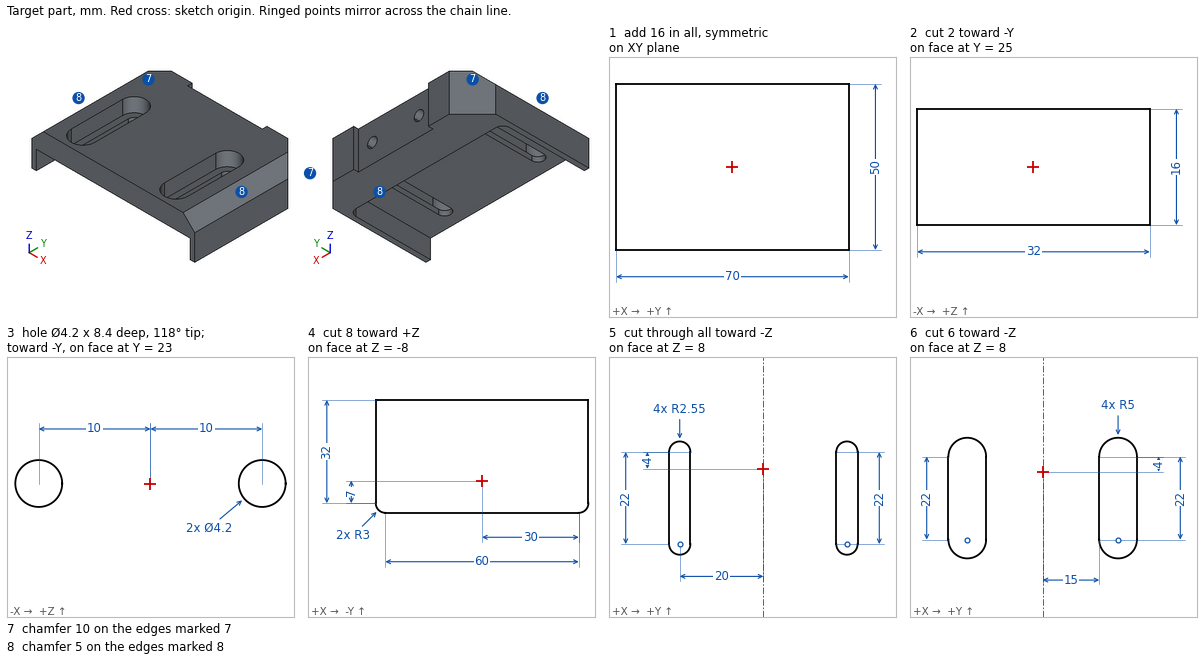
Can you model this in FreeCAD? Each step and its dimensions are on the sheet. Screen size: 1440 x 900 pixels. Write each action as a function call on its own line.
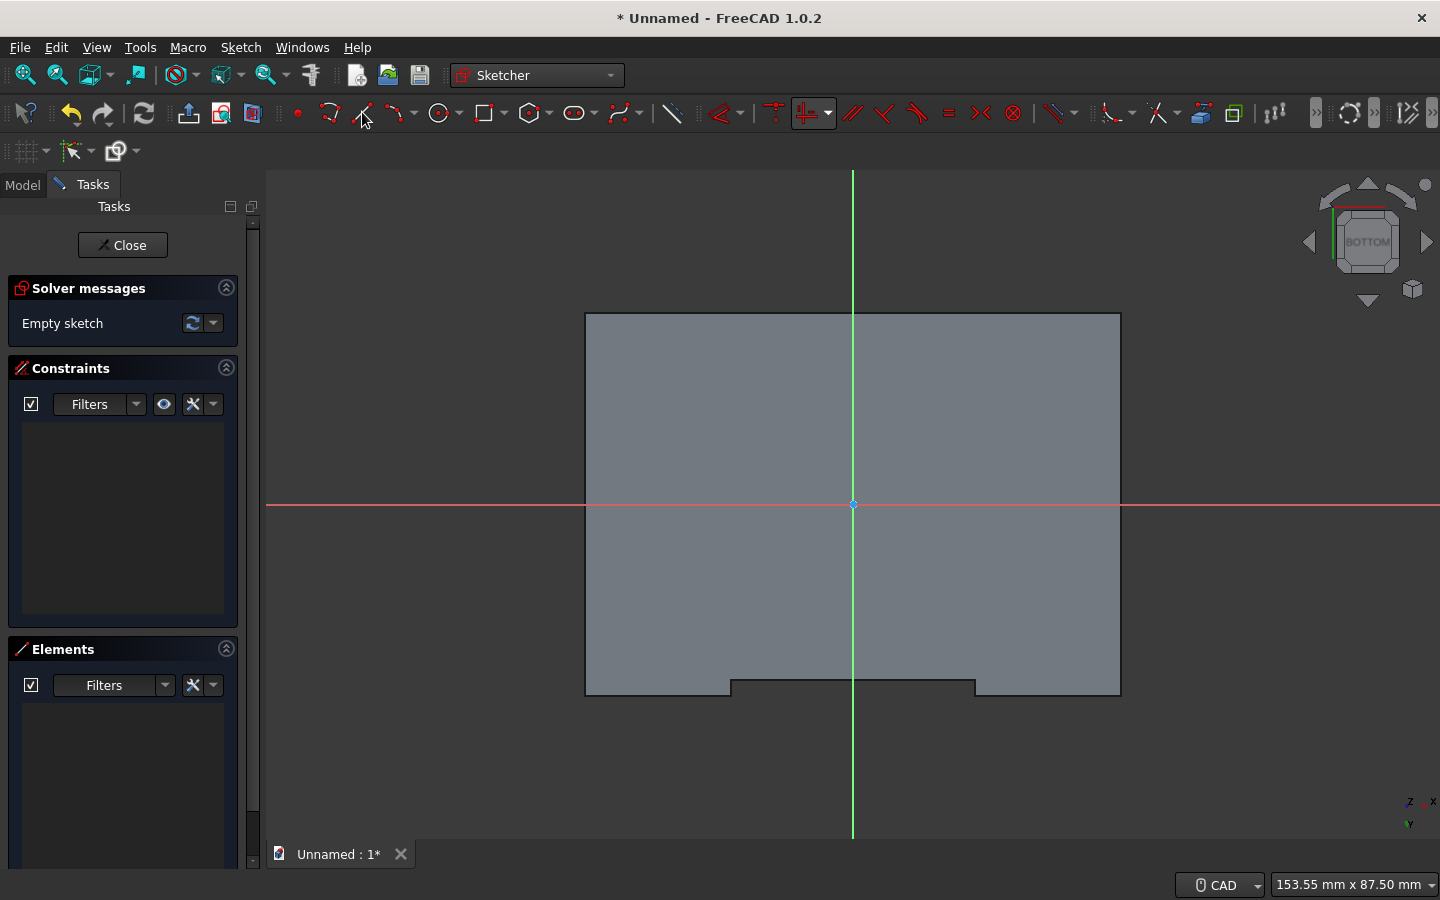
scroll(992, 331, up, 2)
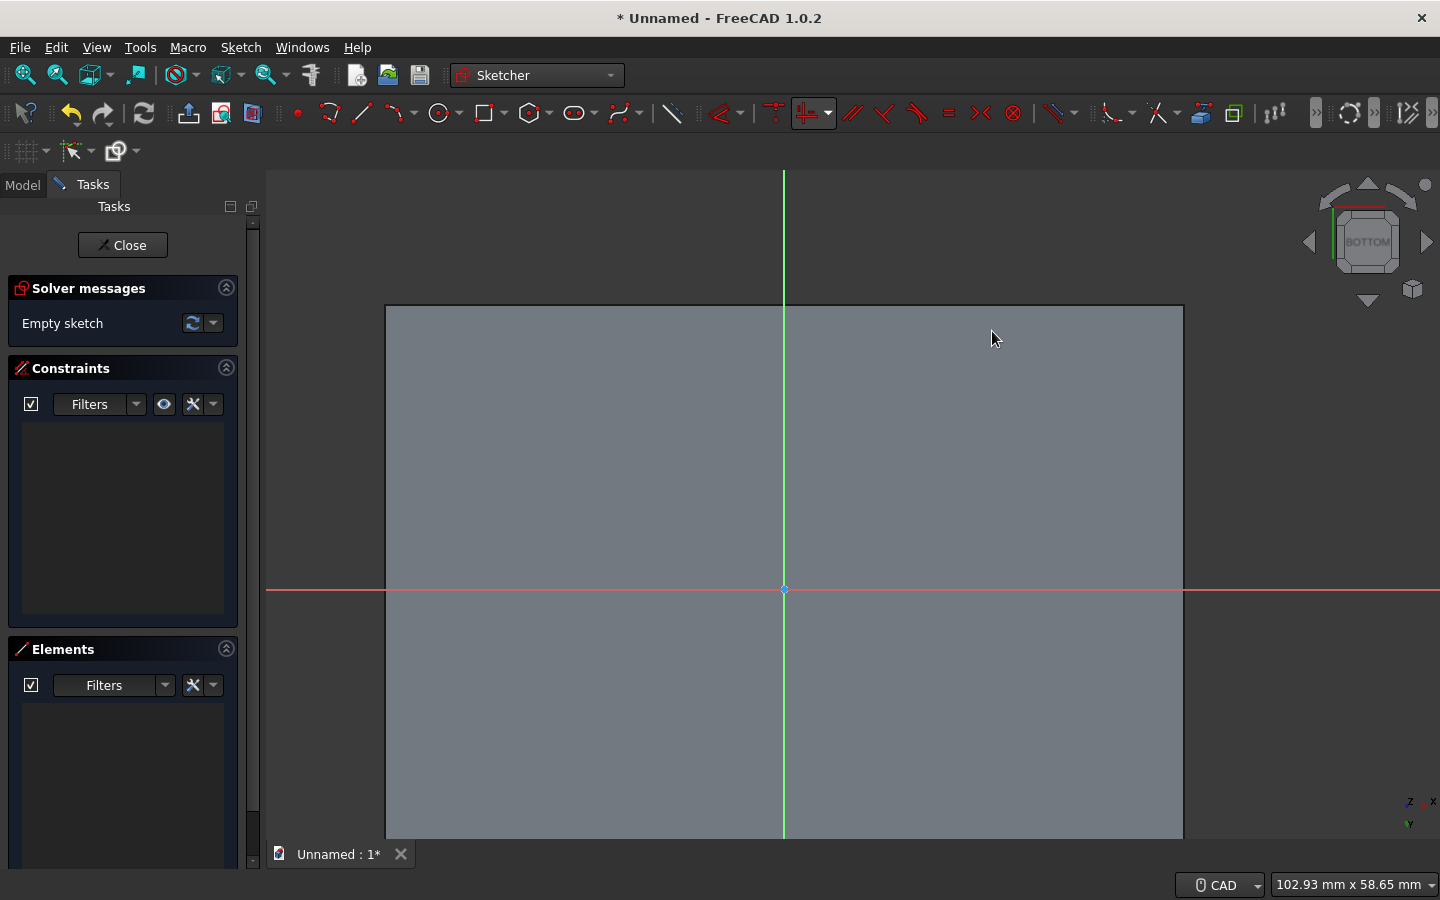
key(g)
key(l)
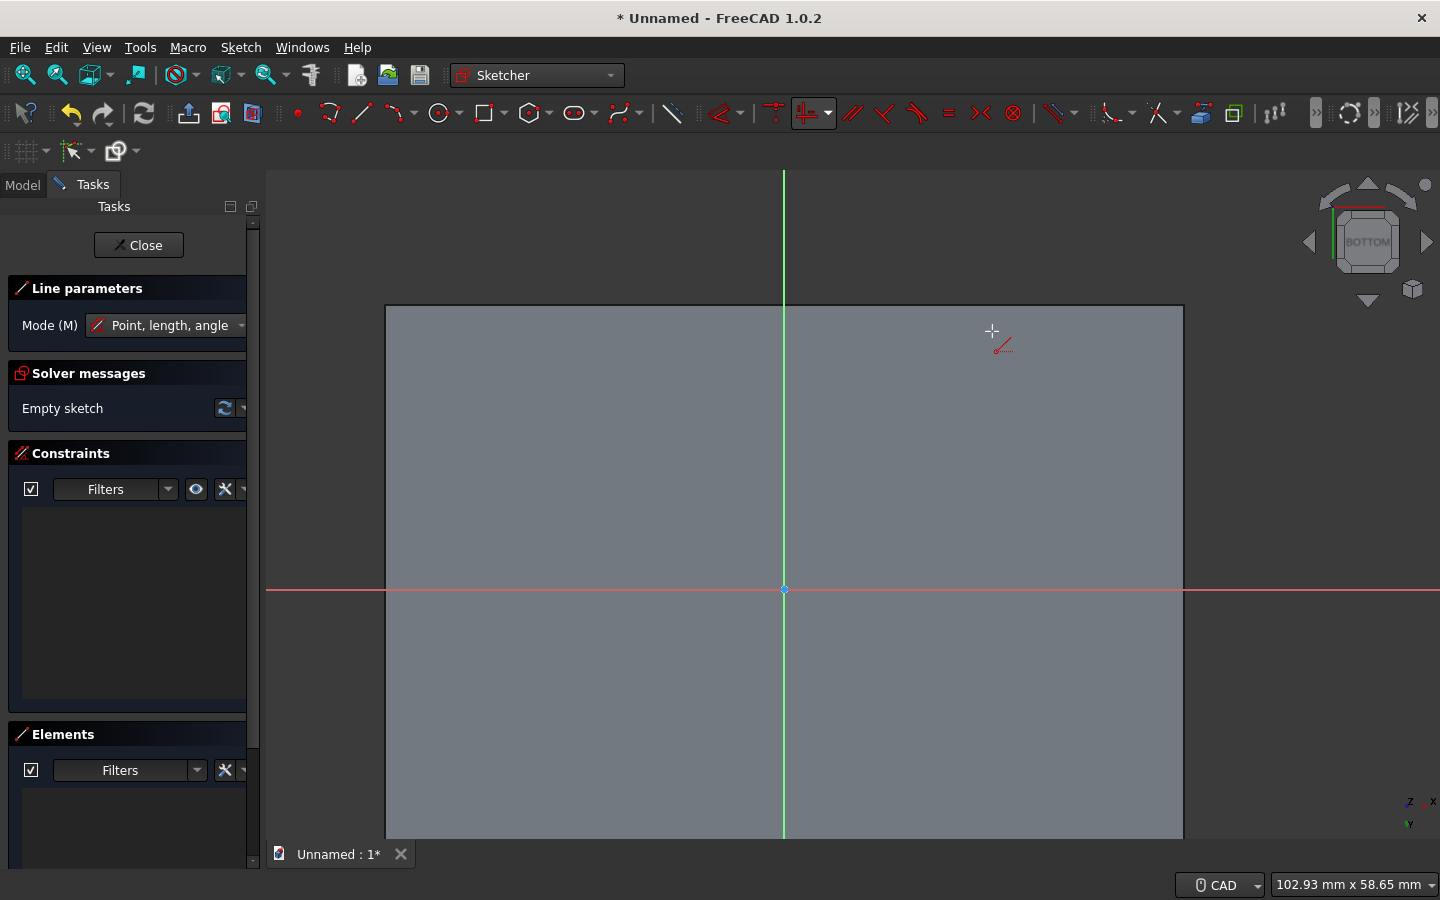
click(1127, 704)
click(442, 704)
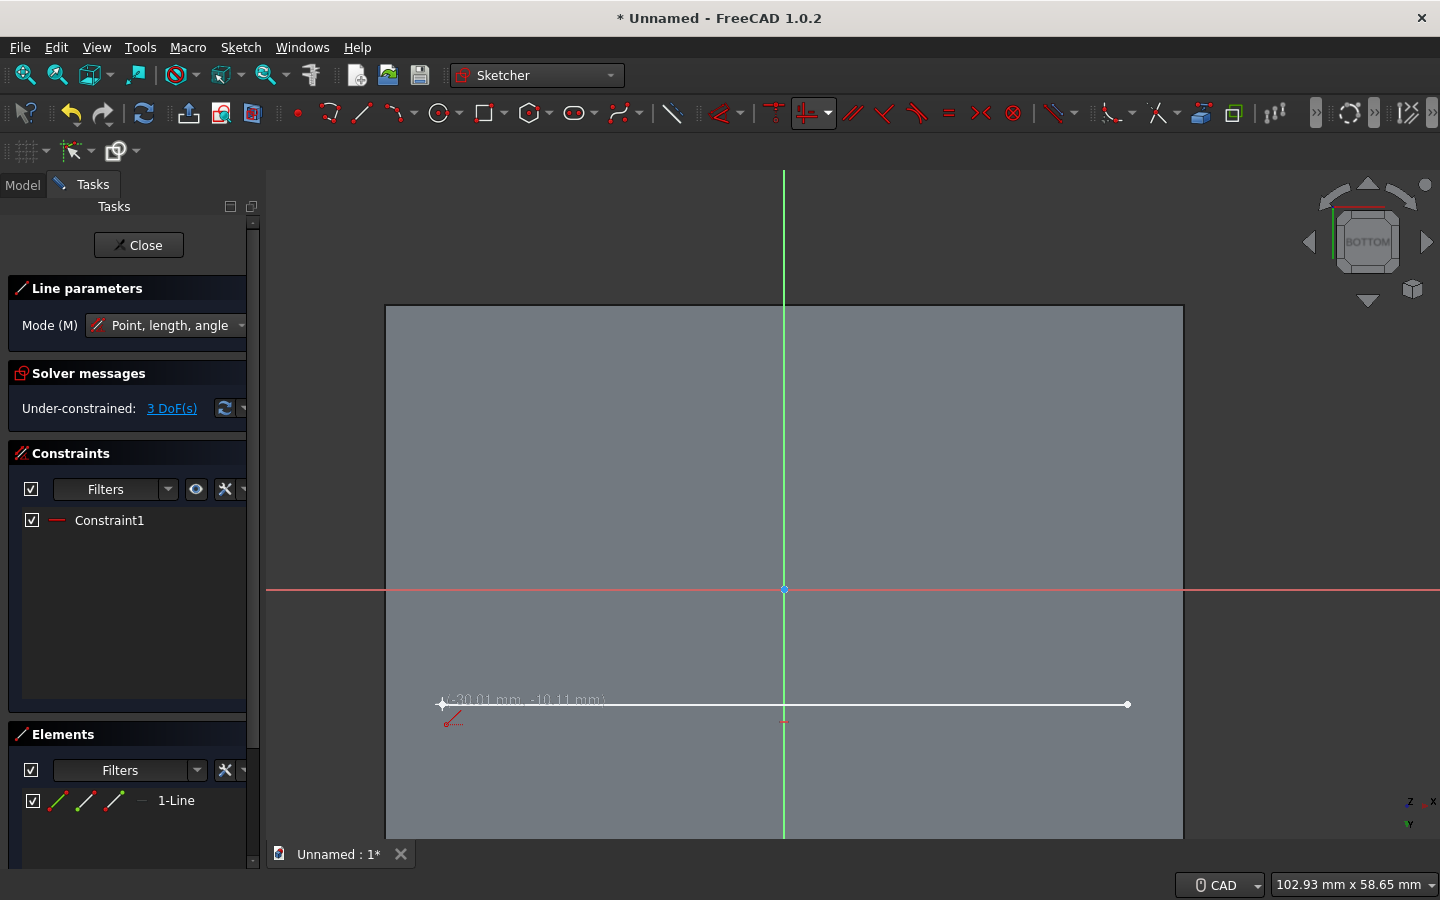
click(330, 114)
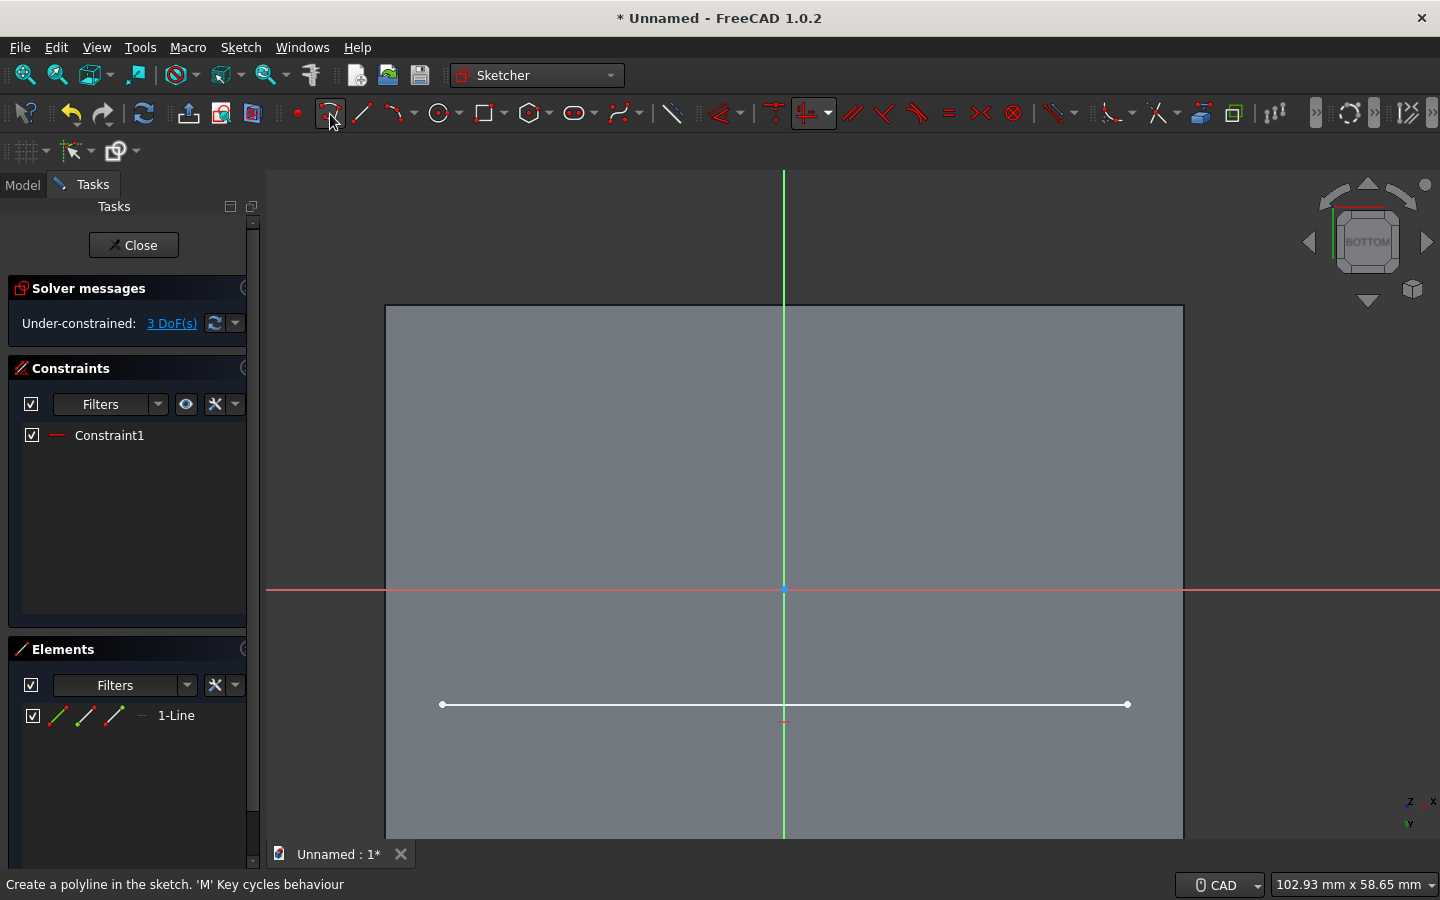
click(408, 670)
click(408, 305)
click(1161, 305)
click(1161, 670)
right_click(1161, 670)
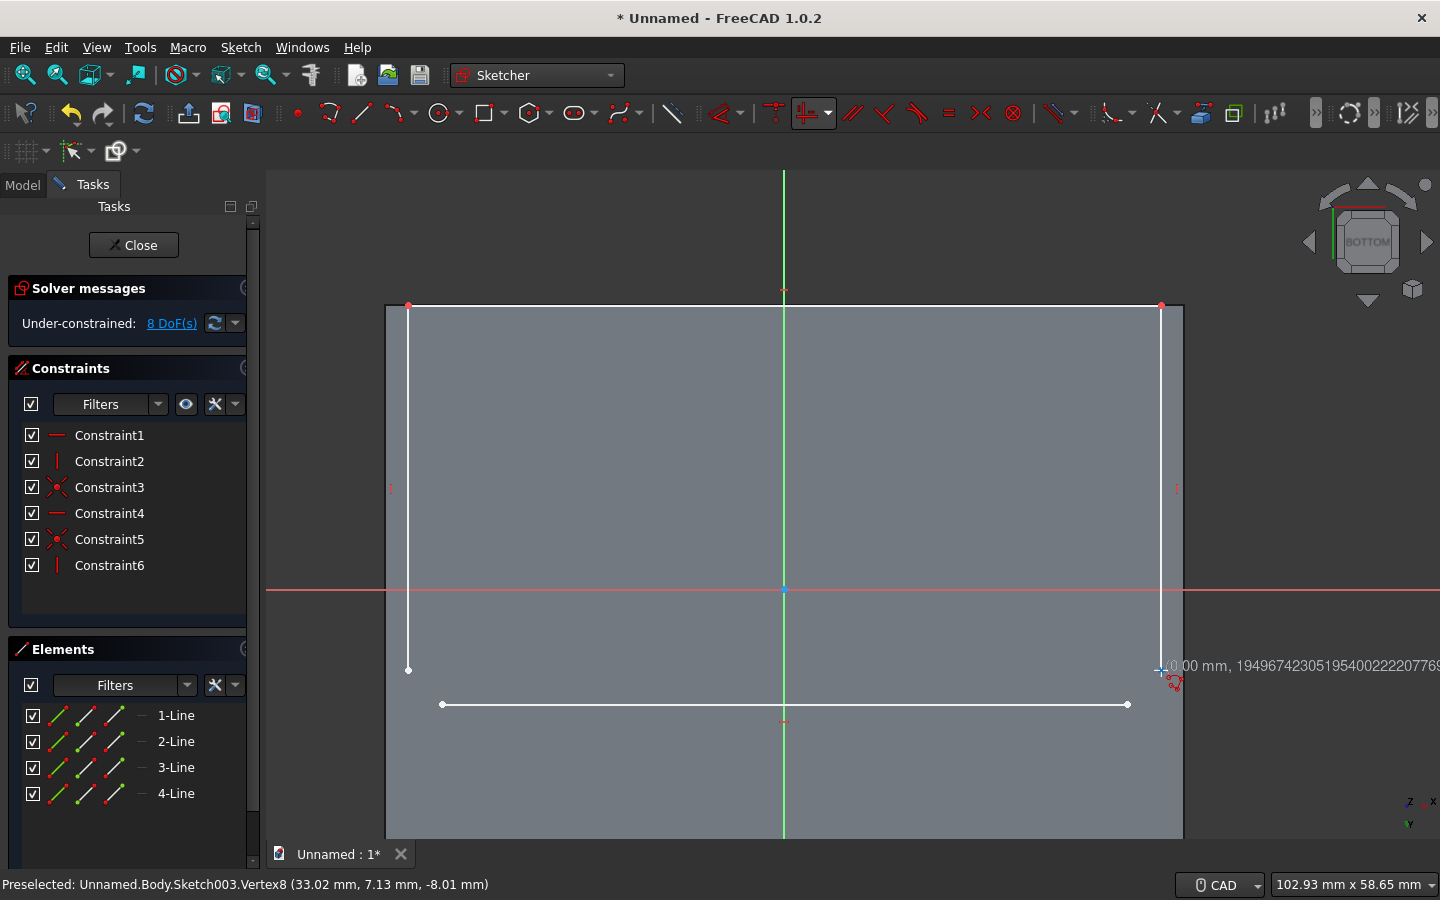
key(g)
key(3)
key(a)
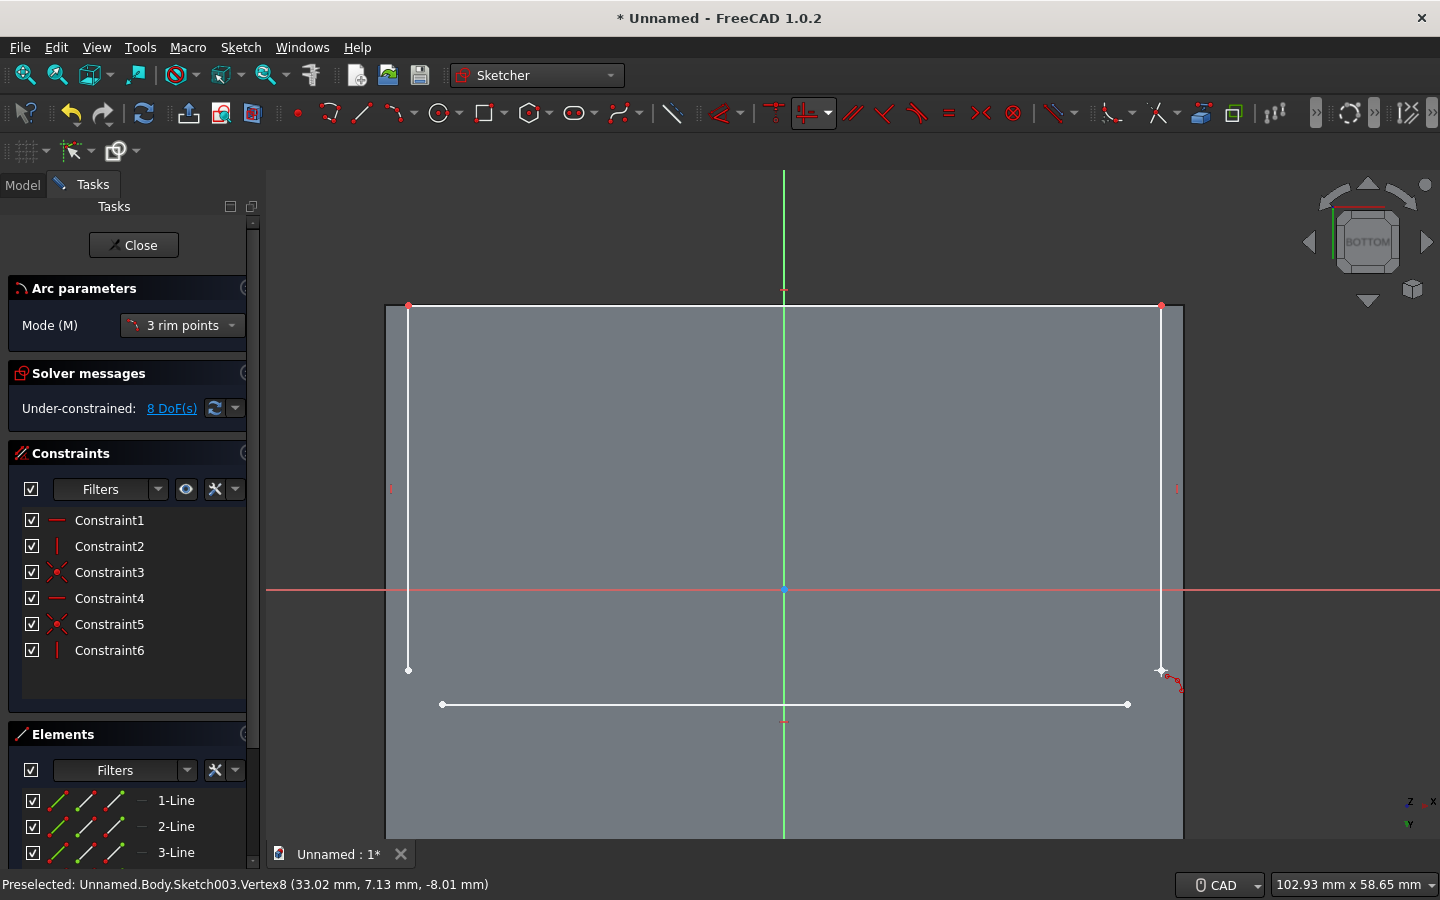
click(442, 705)
click(408, 671)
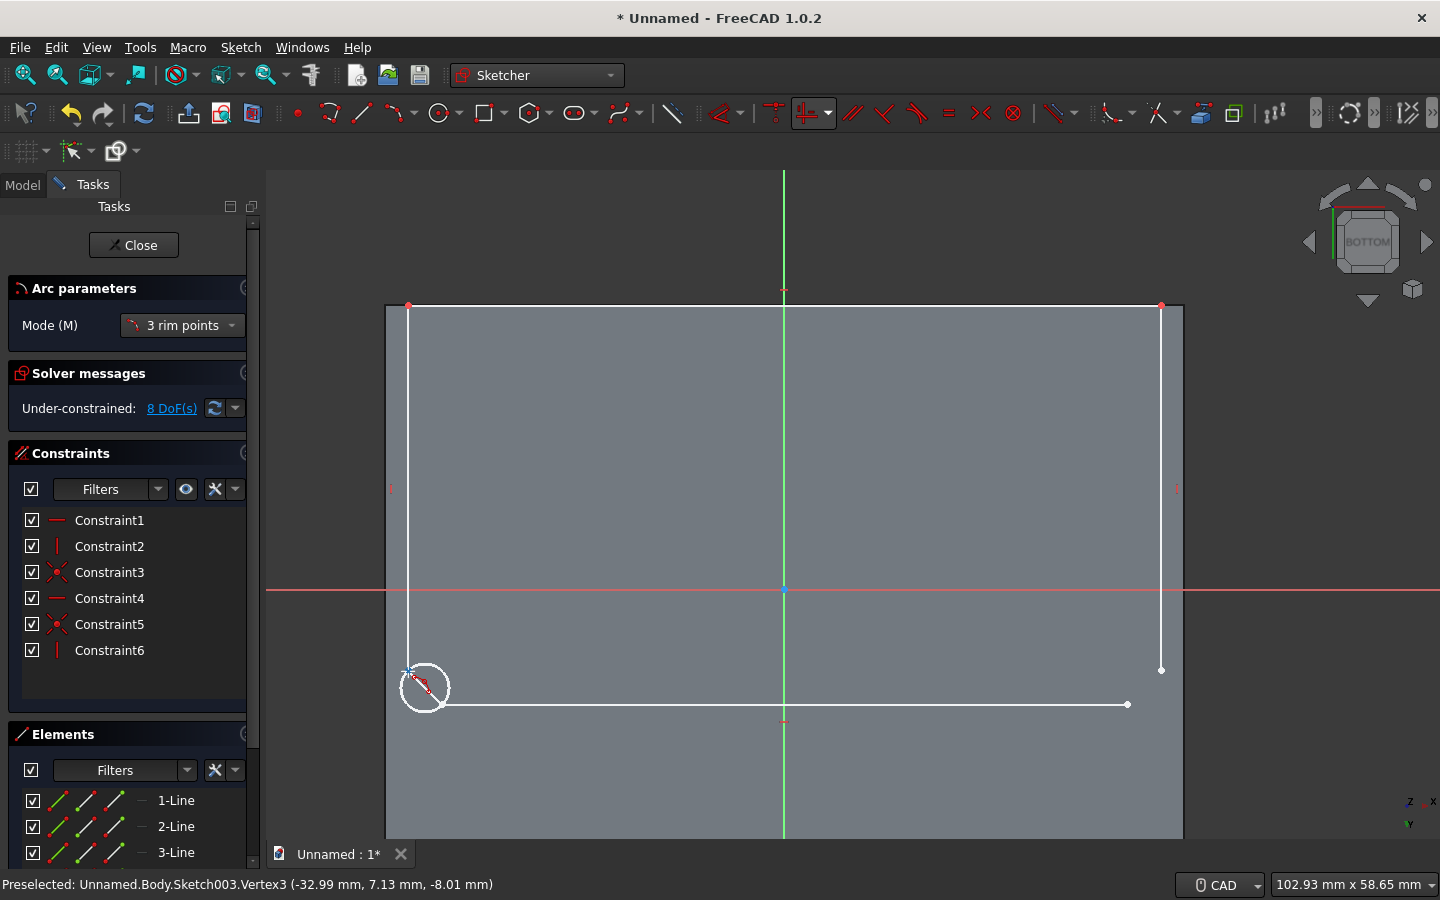
scroll(418, 694, up, 3)